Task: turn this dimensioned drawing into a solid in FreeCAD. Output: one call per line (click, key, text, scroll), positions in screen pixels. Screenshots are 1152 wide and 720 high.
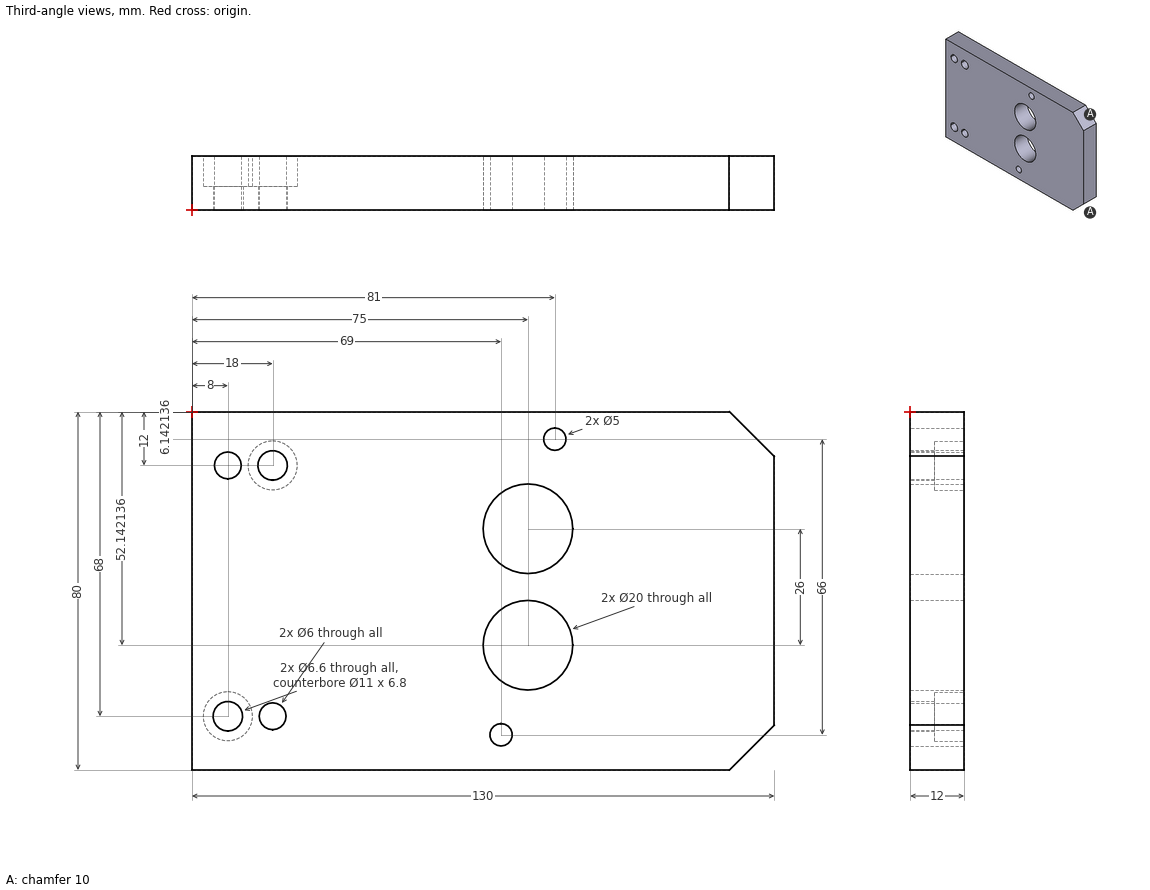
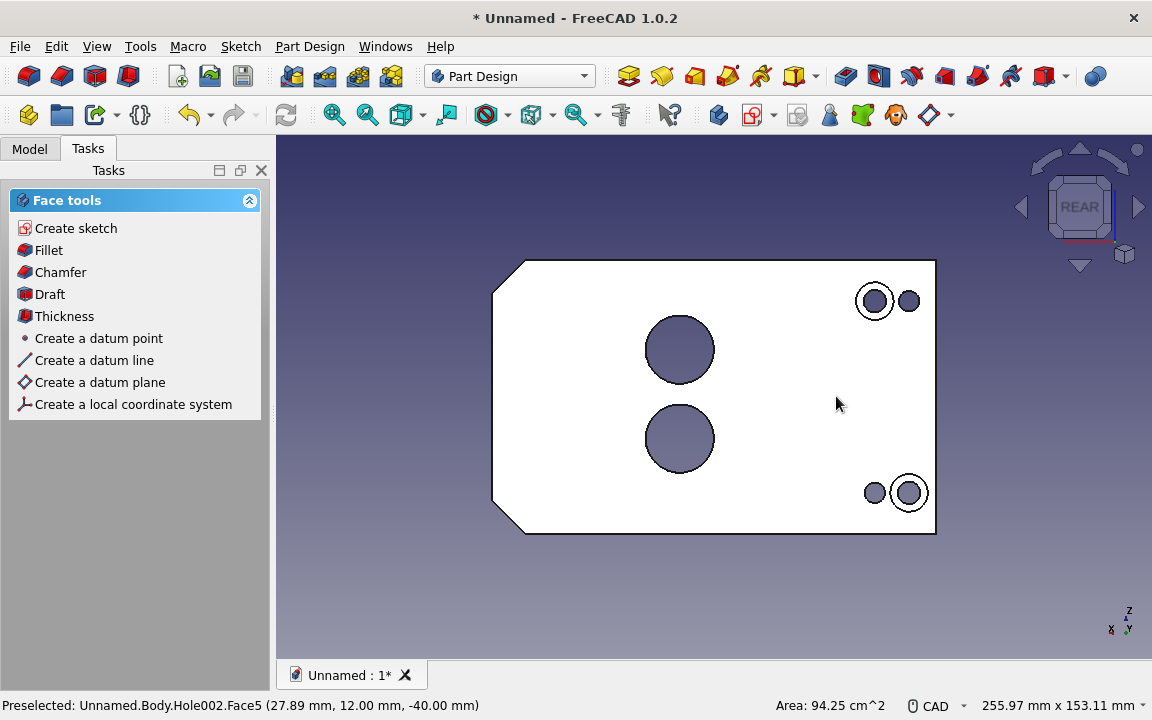
click(752, 116)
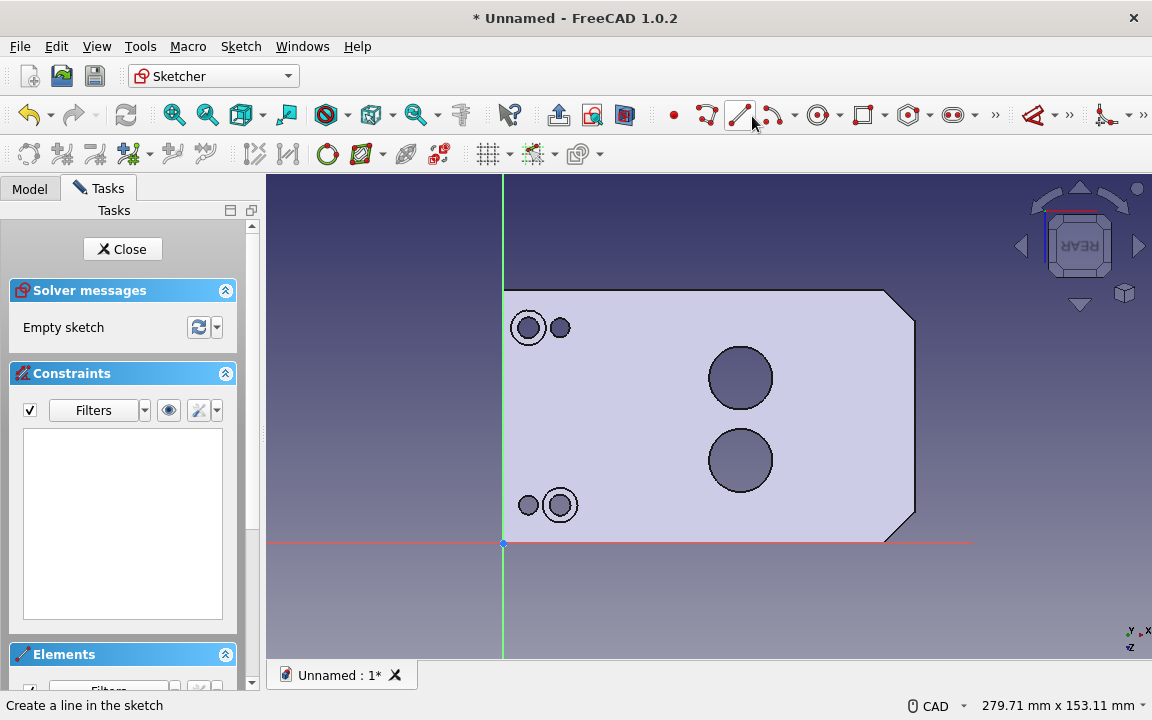
key(g)
key(c)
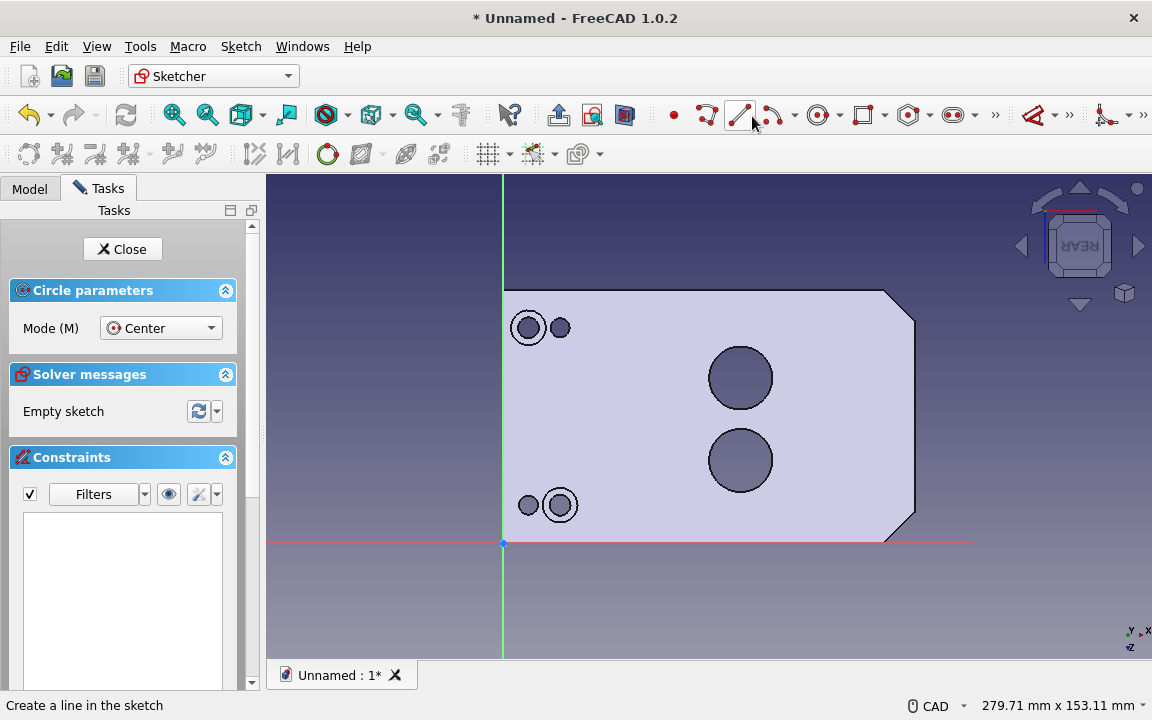
scroll(760, 524, up, 6)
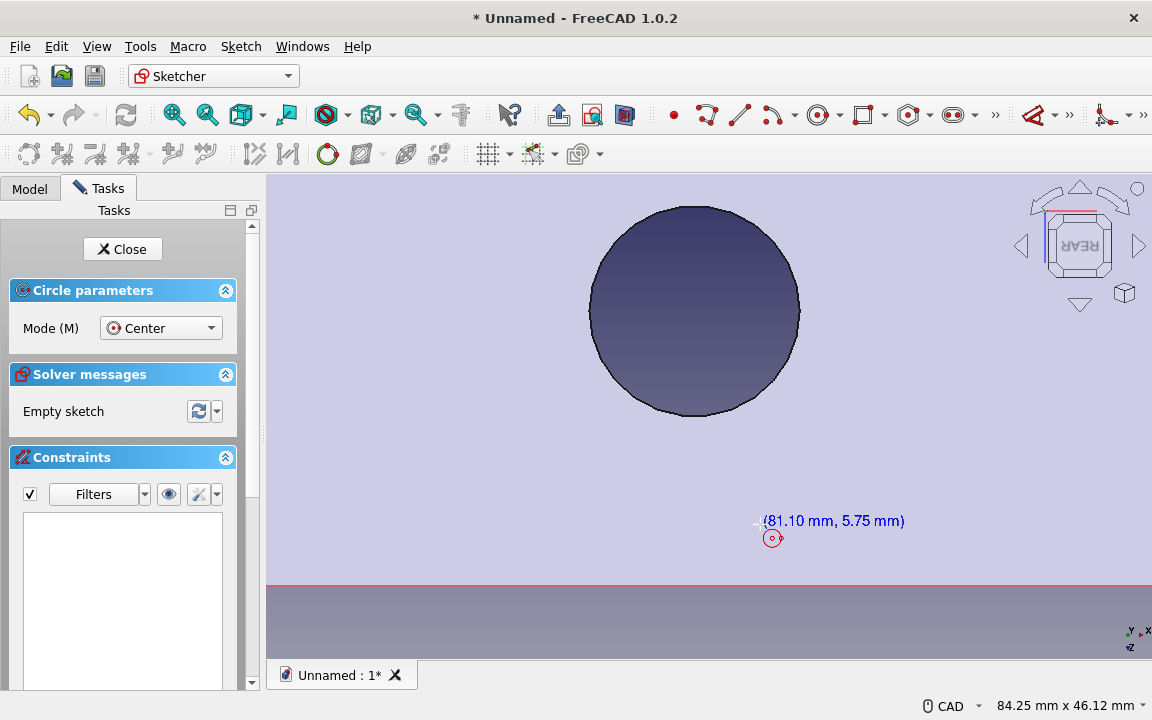
click(758, 521)
click(776, 503)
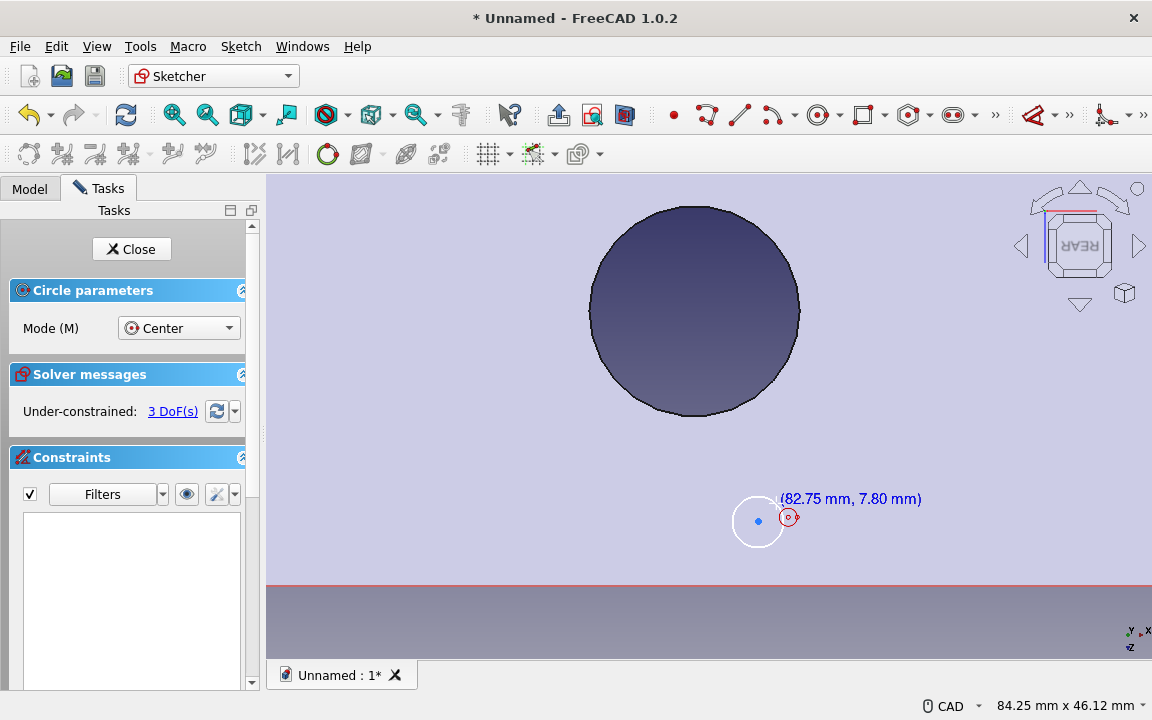
scroll(813, 546, down, 5)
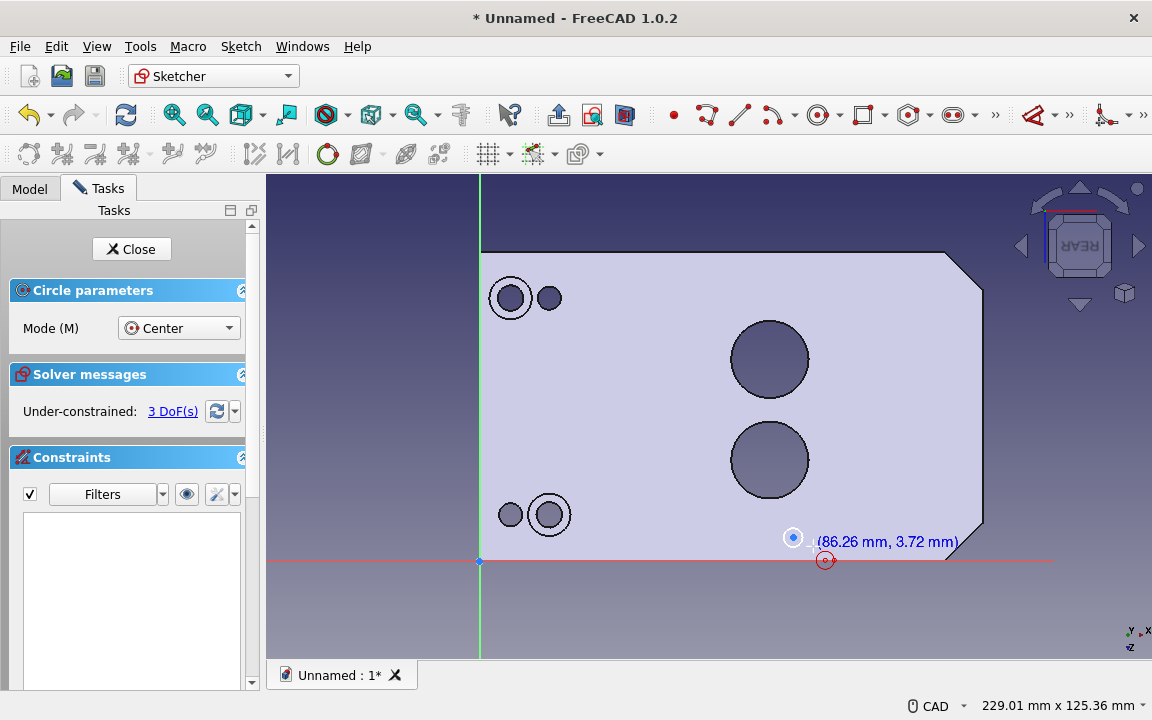
scroll(747, 282, up, 5)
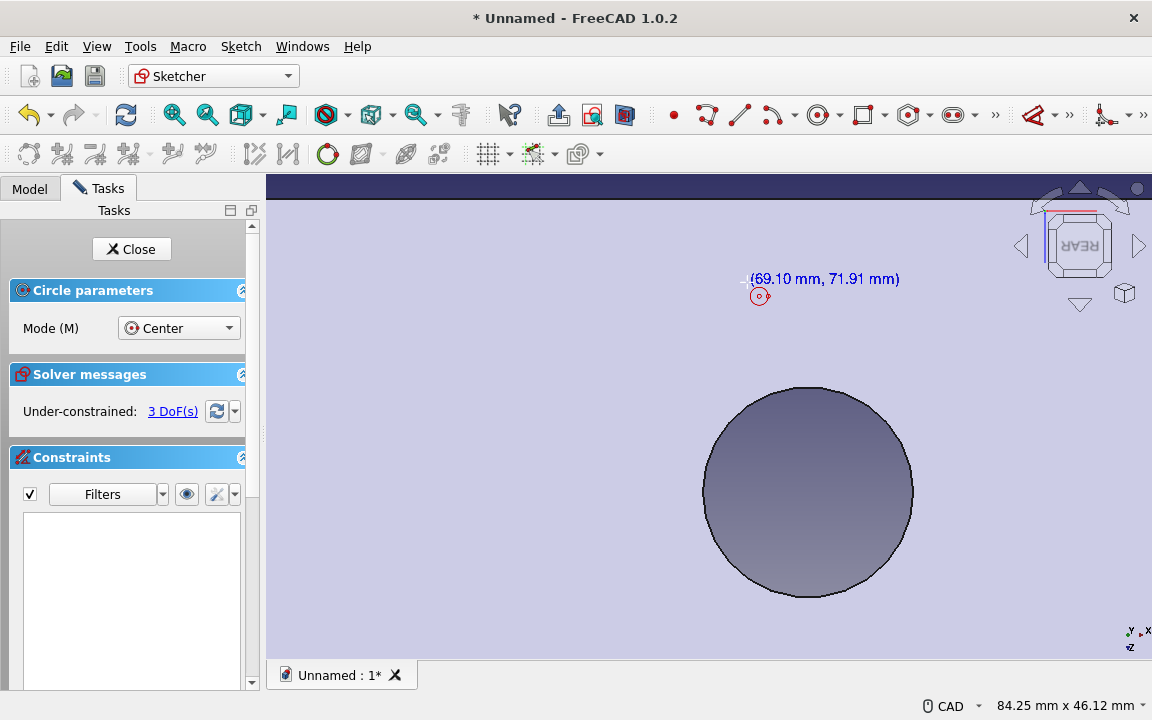
click(745, 282)
click(764, 263)
key(Escape)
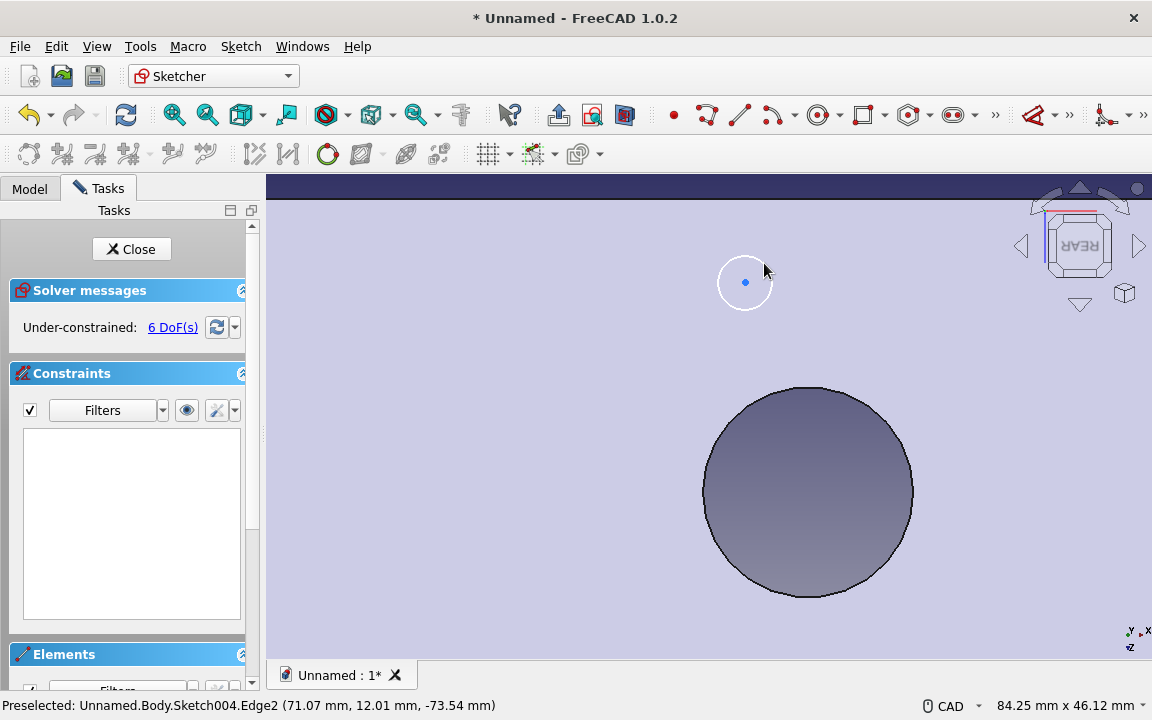
scroll(746, 282, down, 5)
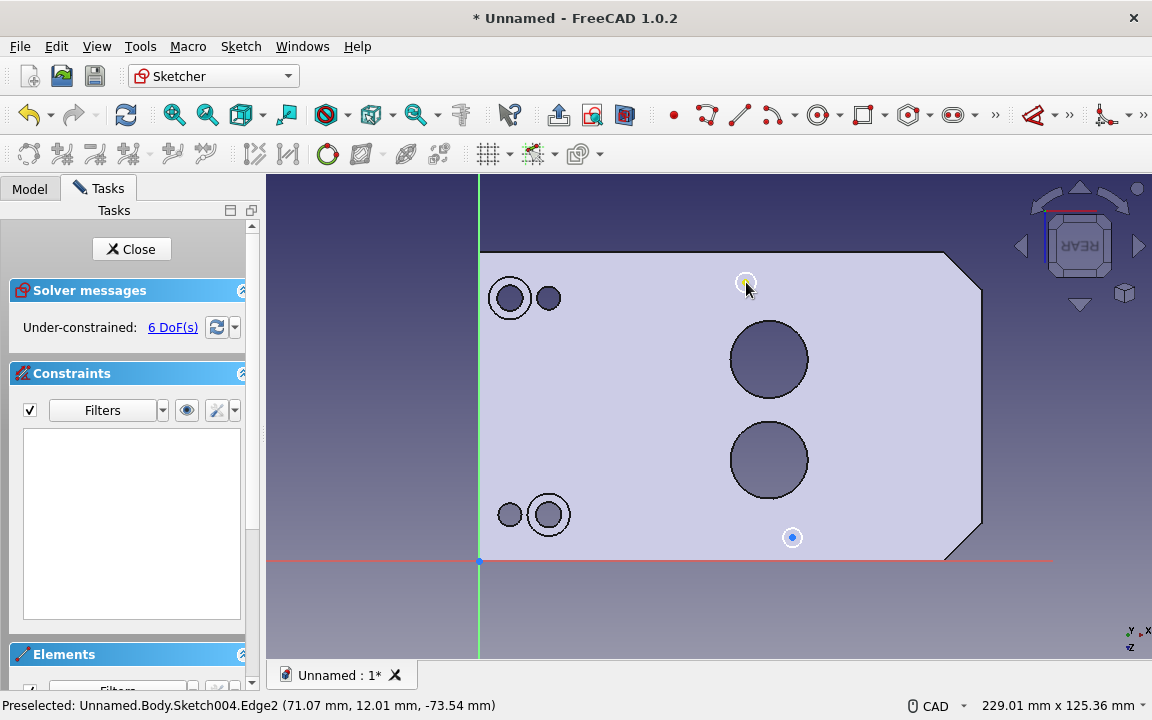
scroll(799, 531, up, 2)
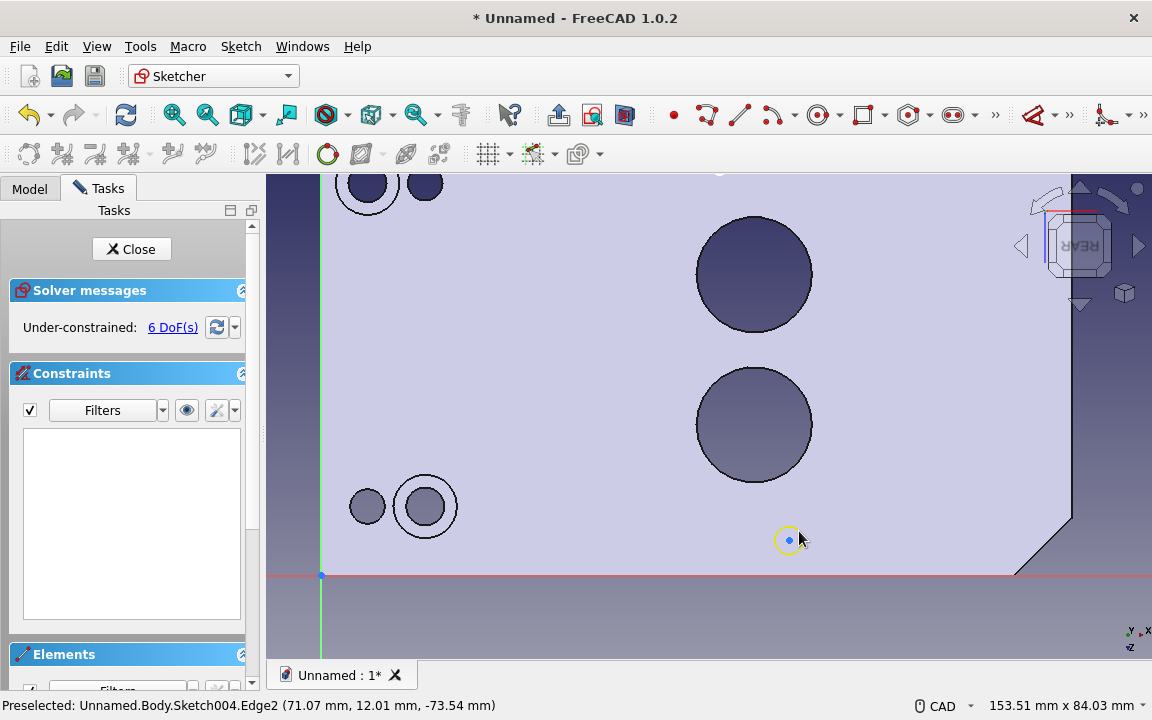
click(799, 531)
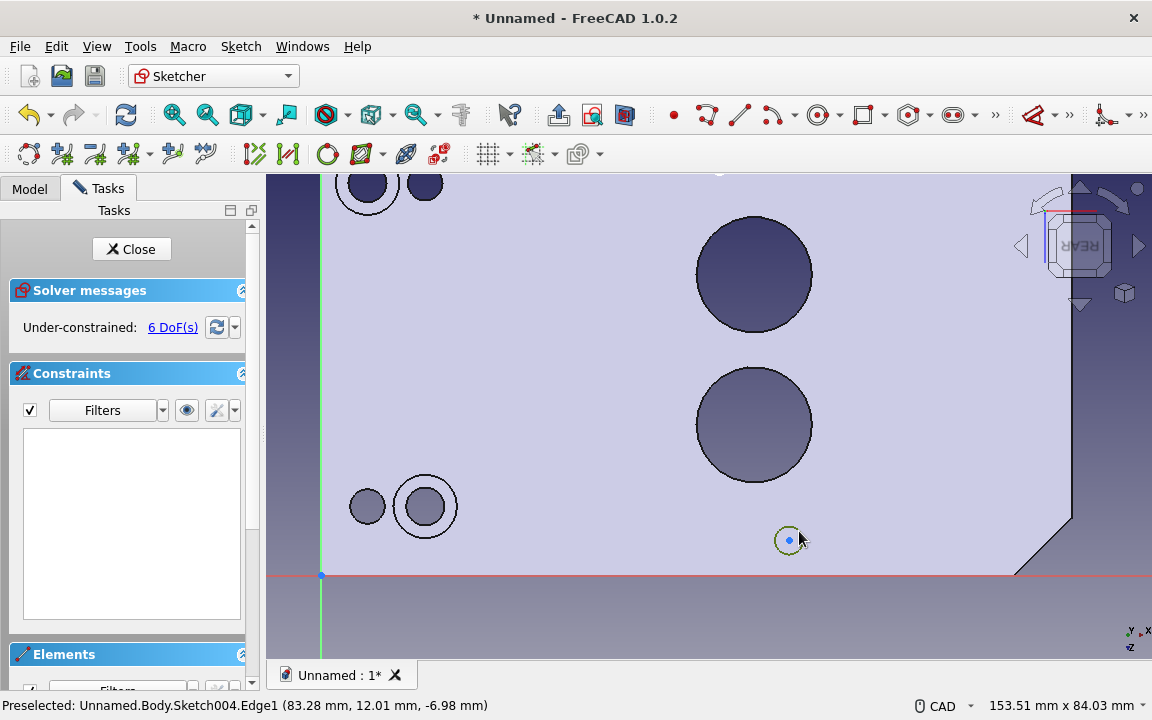
scroll(799, 531, down, 2)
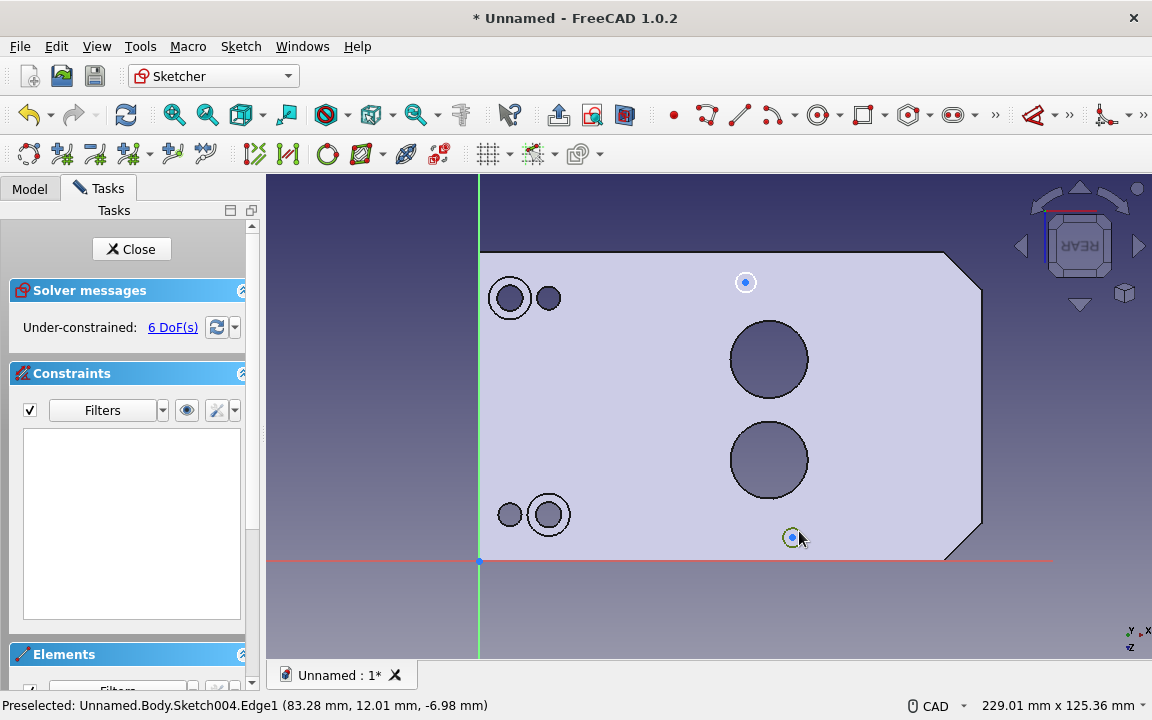
scroll(753, 275, up, 2)